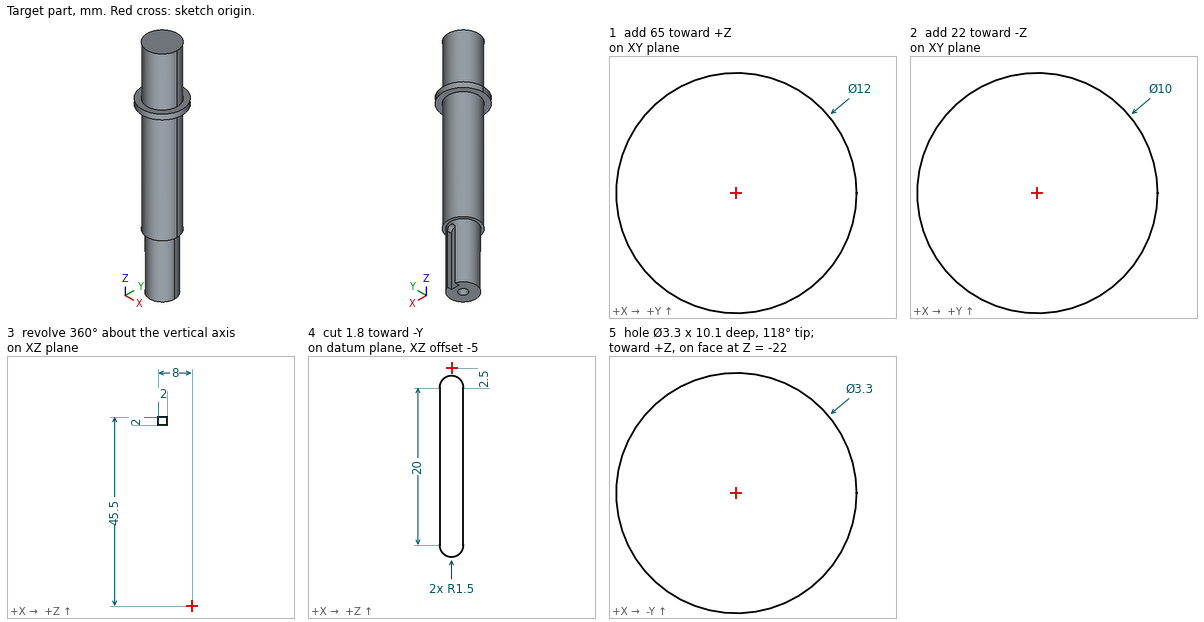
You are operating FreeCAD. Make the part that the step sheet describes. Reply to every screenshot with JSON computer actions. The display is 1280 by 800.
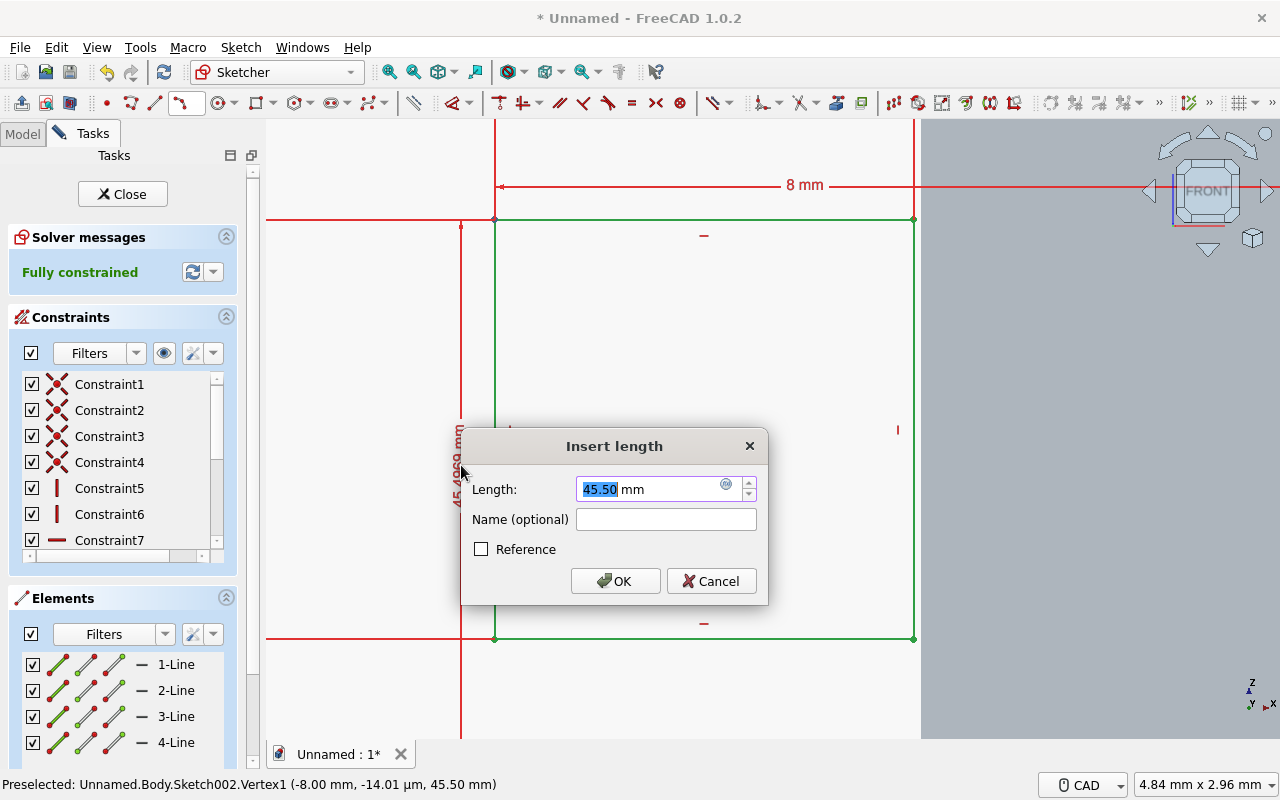
{"action": "type", "text": "45.5"}
{"action": "key", "text": "Return"}
{"action": "key", "text": "Escape"}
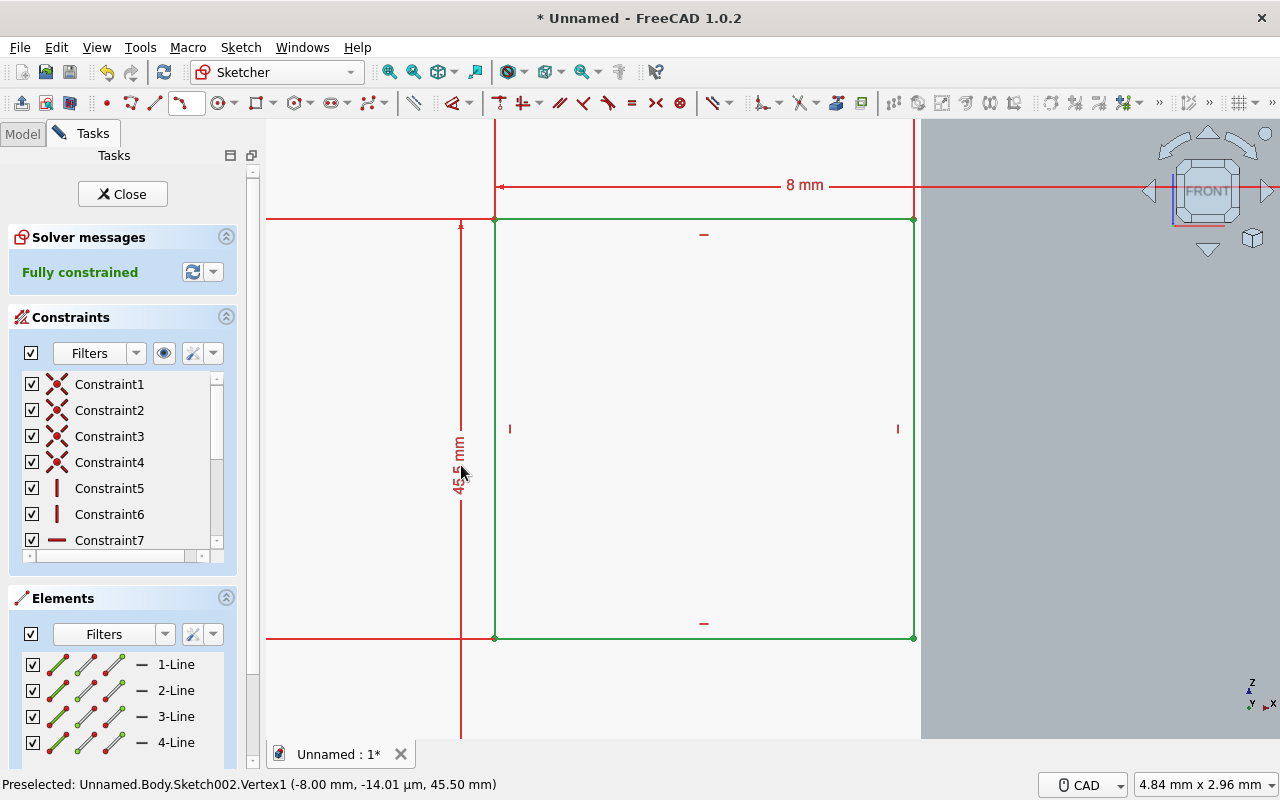
{"action": "left_click", "coordinate": [123, 194]}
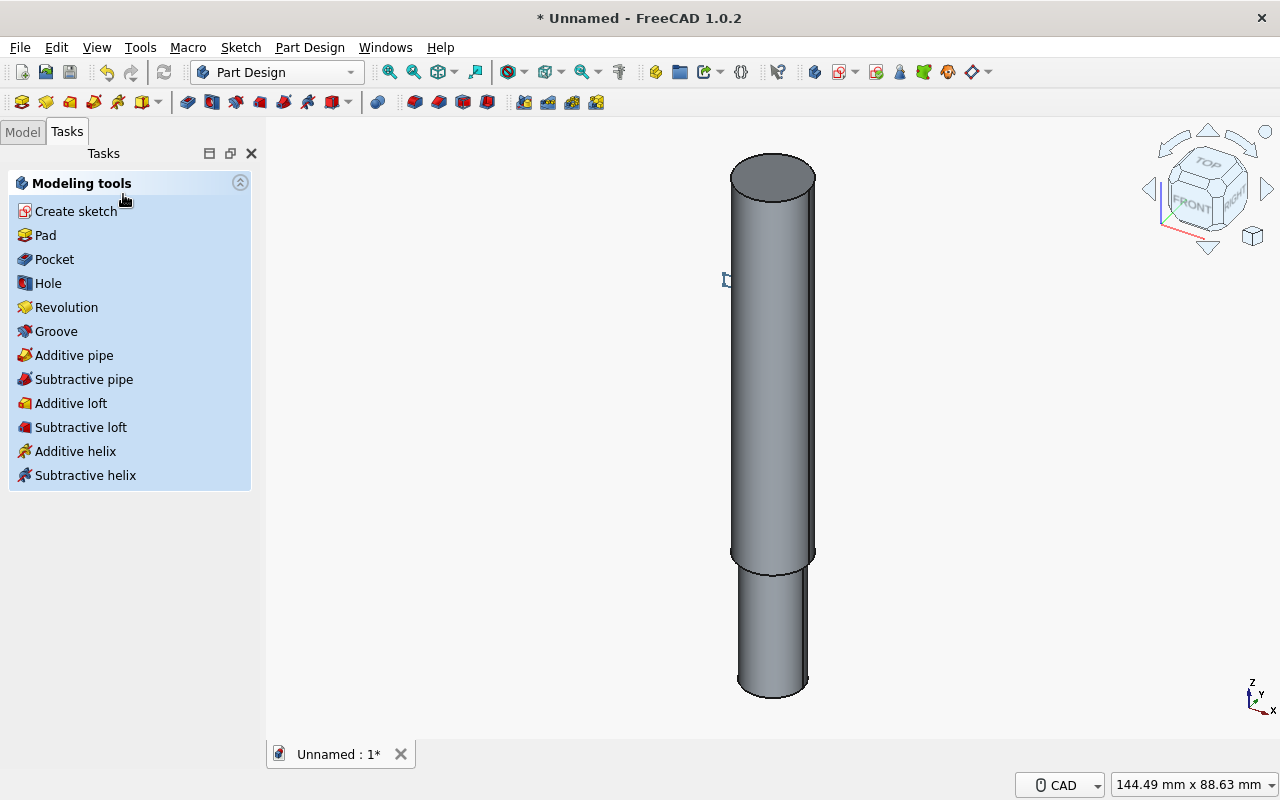
{"action": "left_click", "coordinate": [46, 102]}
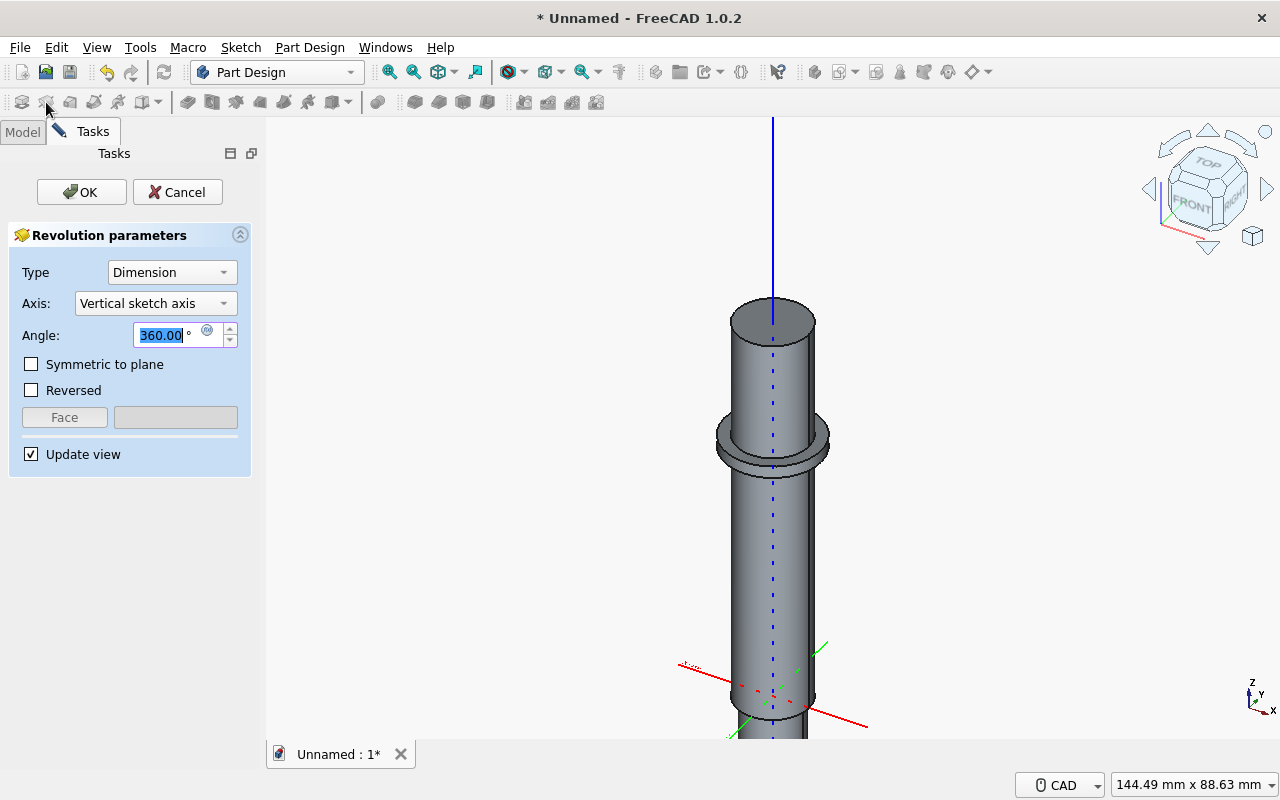
{"action": "left_click", "coordinate": [82, 192]}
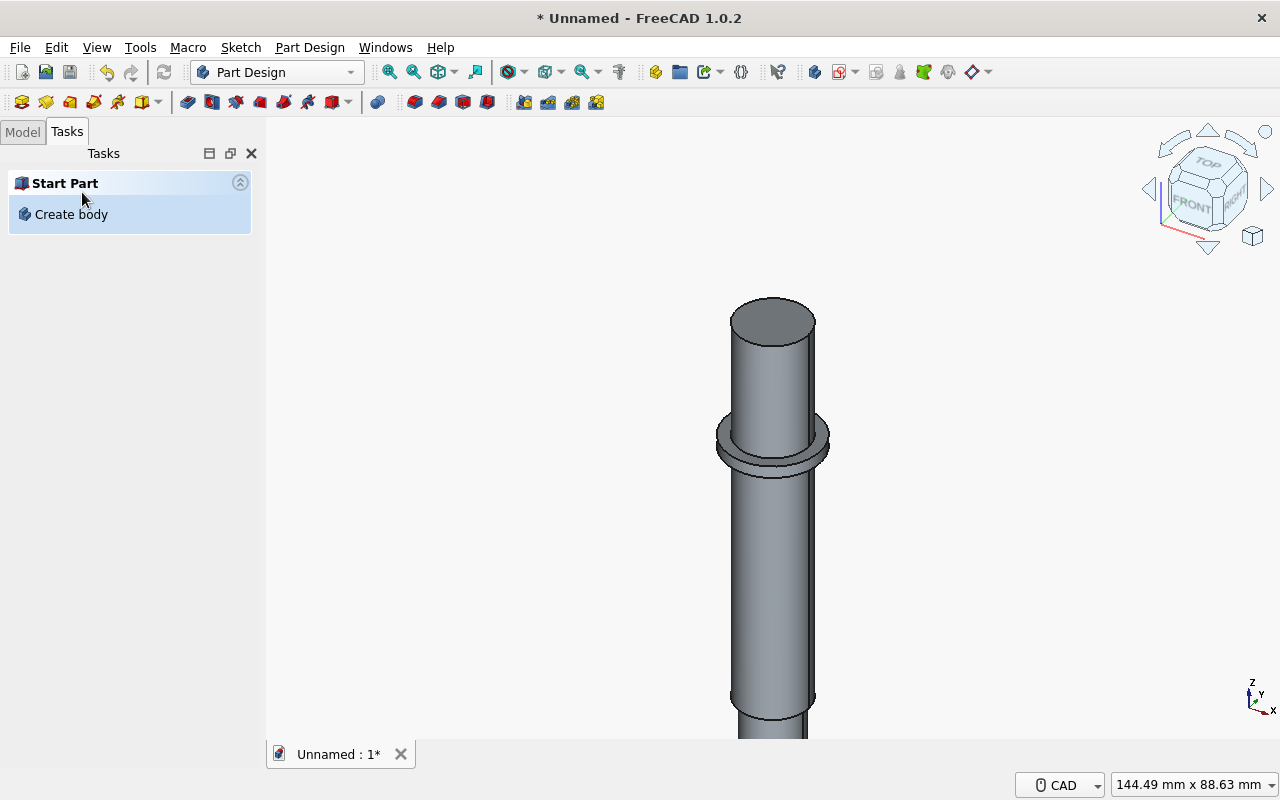
{"action": "left_click", "coordinate": [390, 72]}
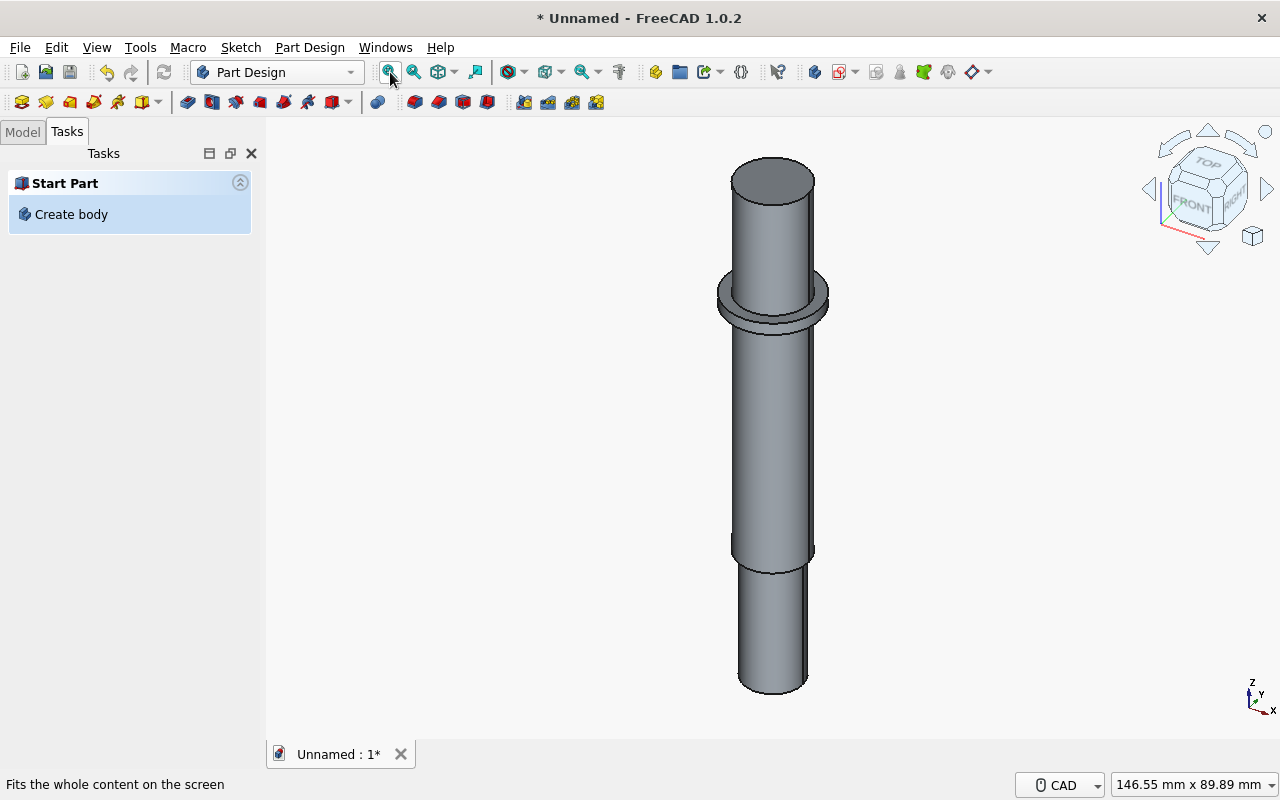
{"action": "left_click", "coordinate": [23, 131]}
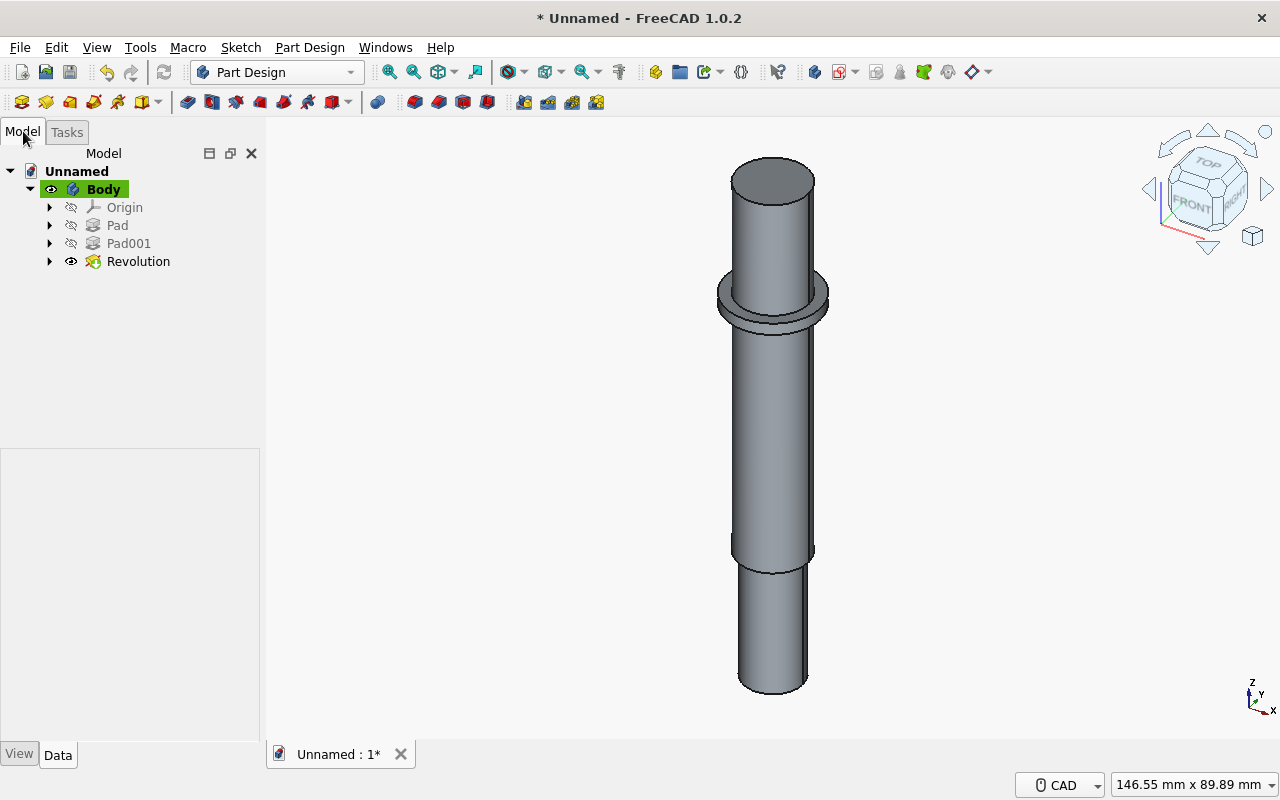
{"action": "left_click", "coordinate": [50, 207]}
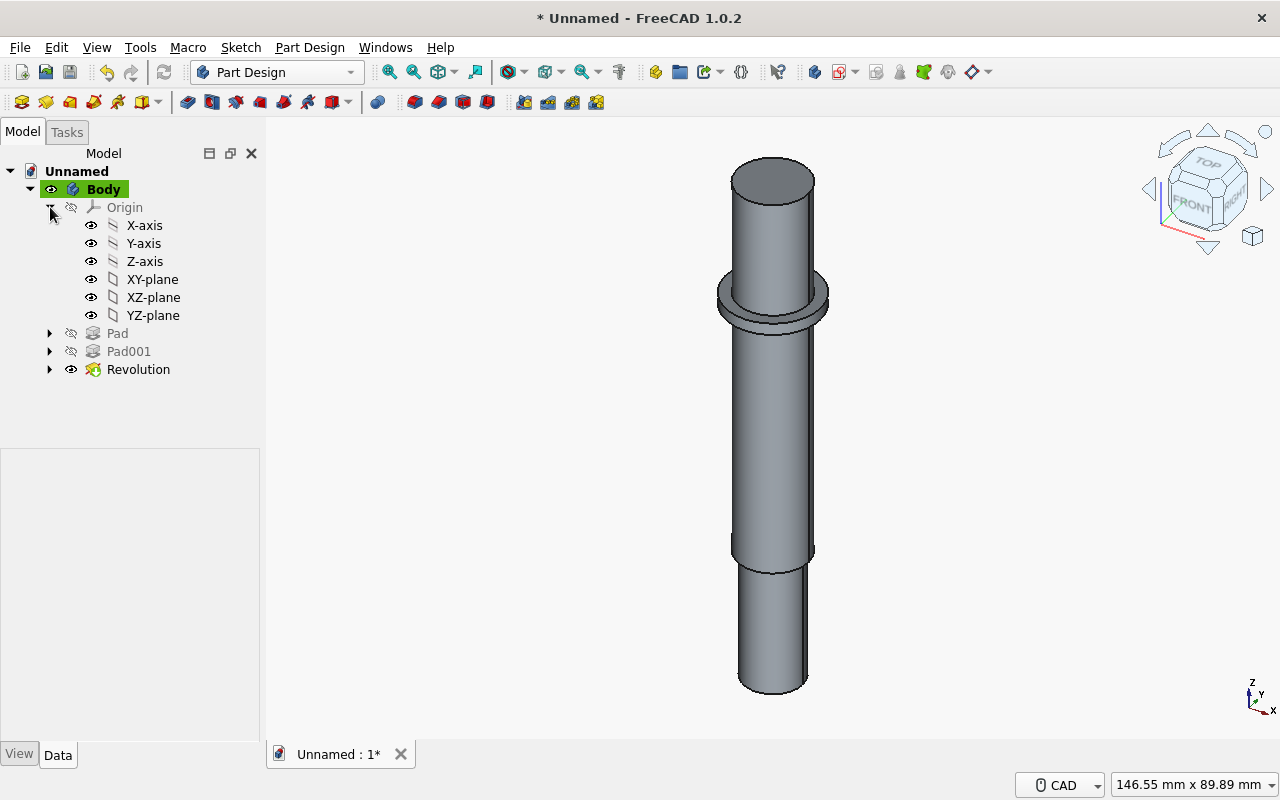
{"action": "left_click", "coordinate": [136, 297]}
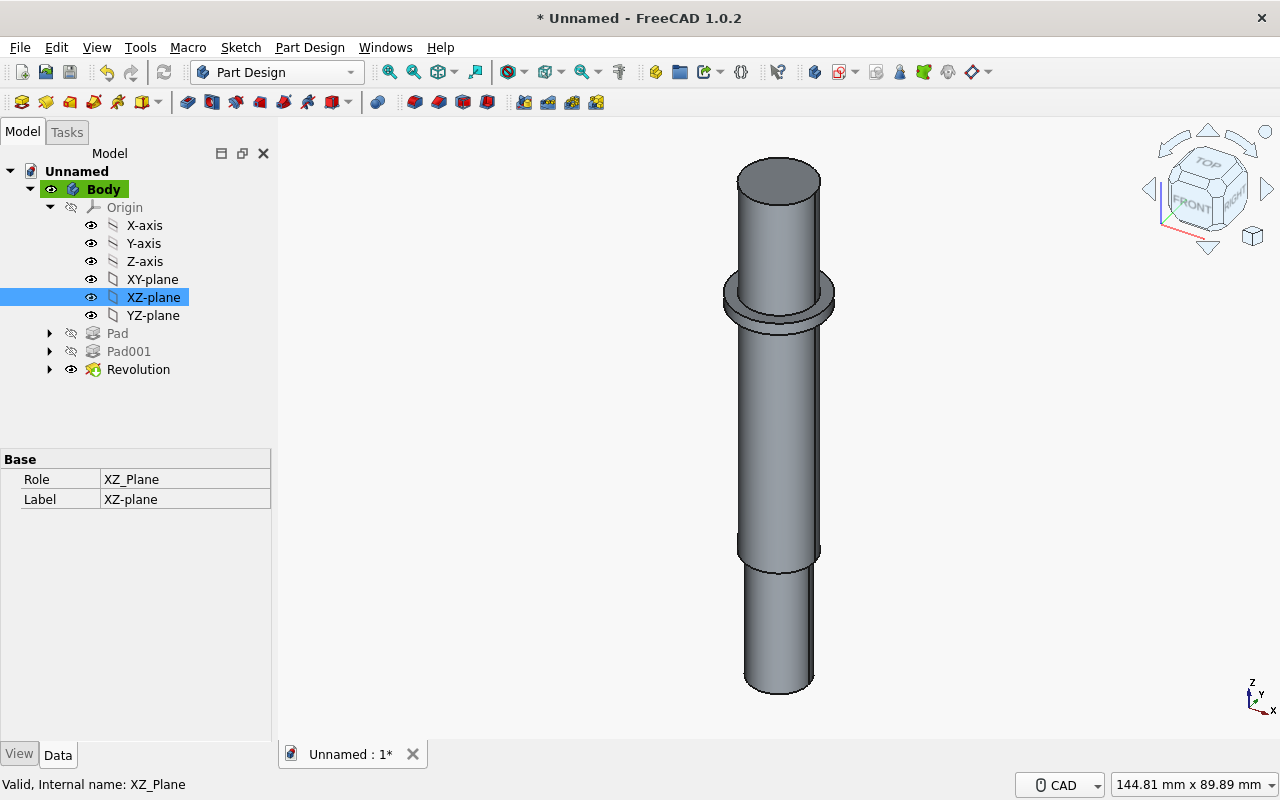
{"action": "left_click", "coordinate": [972, 72]}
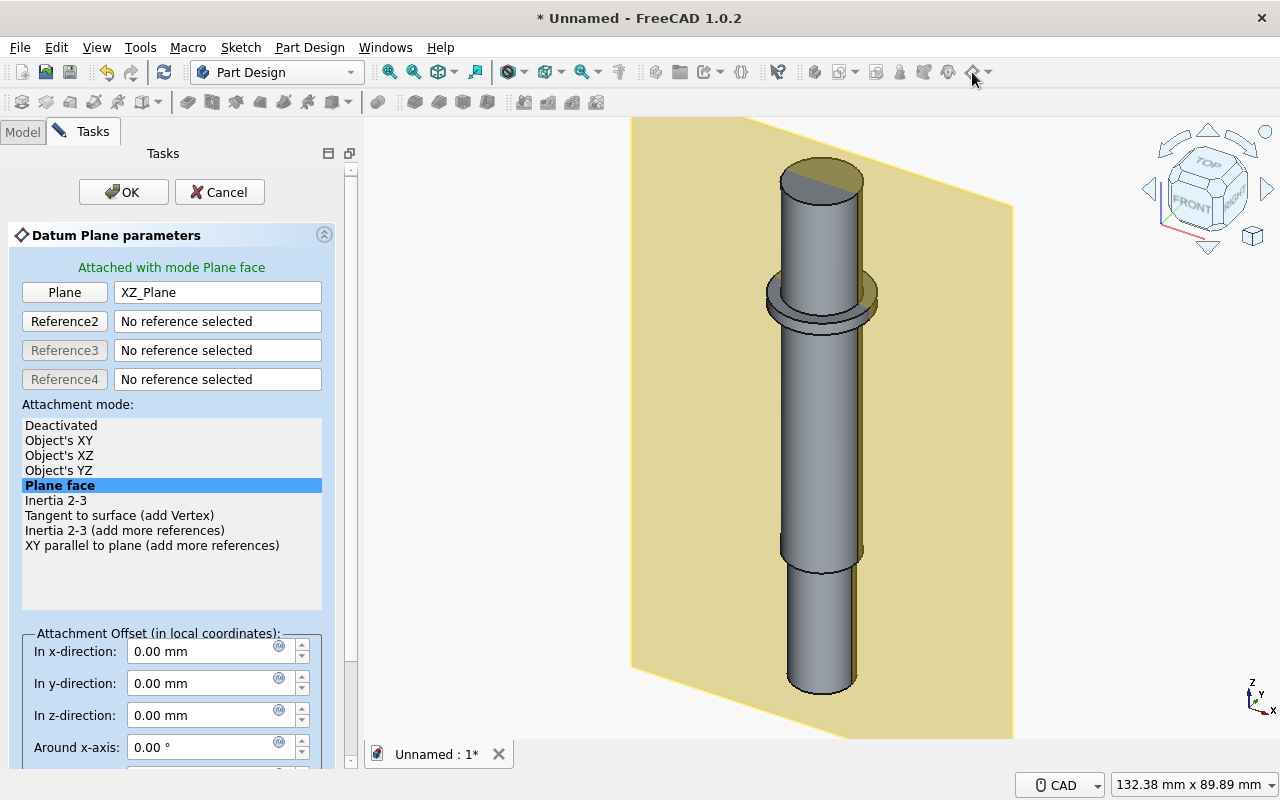
{"action": "triple_click", "coordinate": [210, 715]}